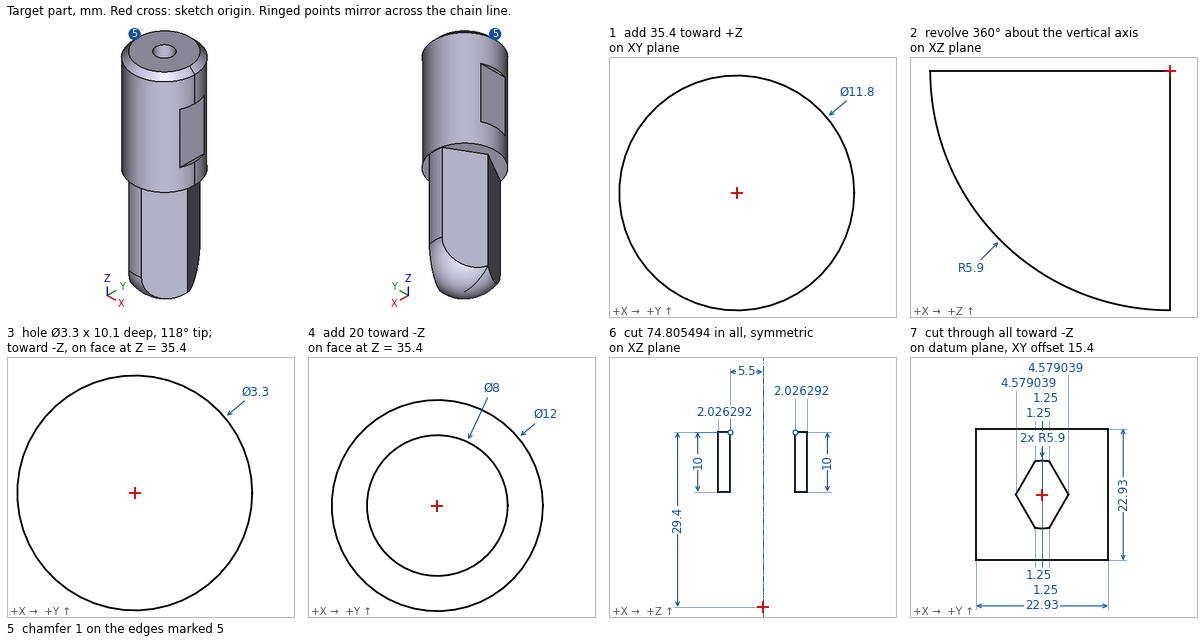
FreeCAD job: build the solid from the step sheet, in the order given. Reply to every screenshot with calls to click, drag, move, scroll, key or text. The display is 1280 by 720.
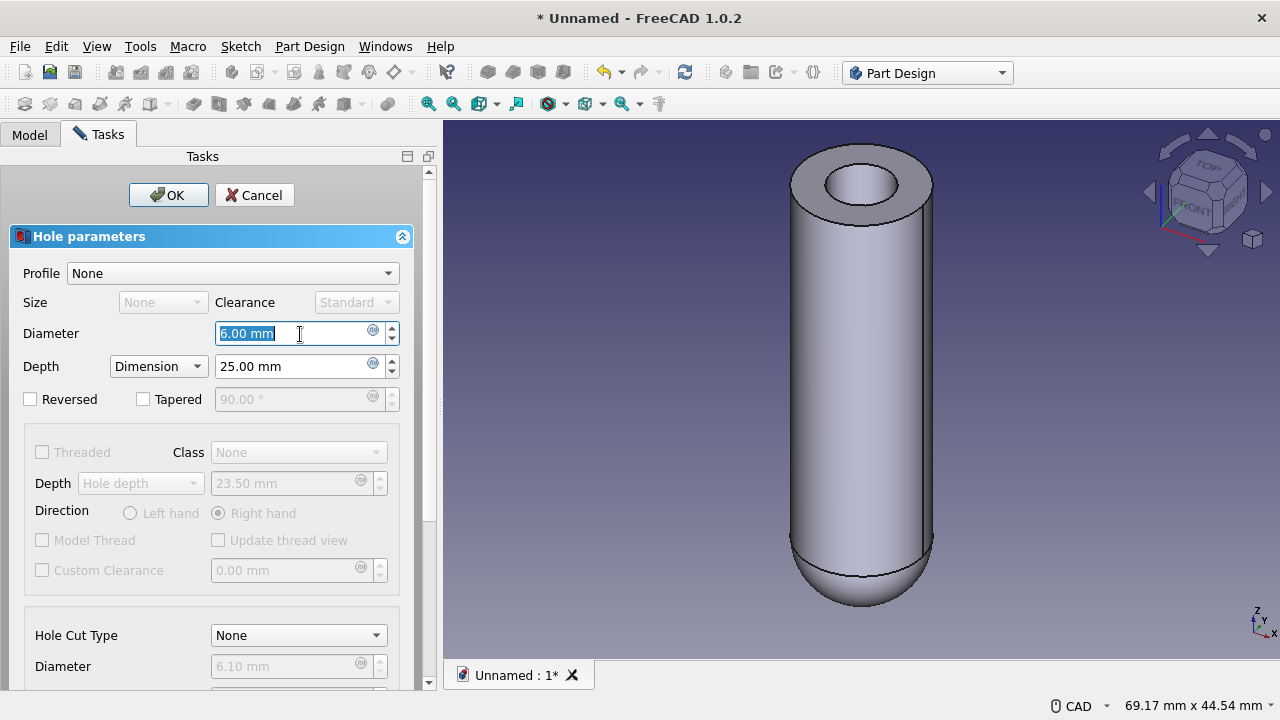
text(3.3)
key(Tab)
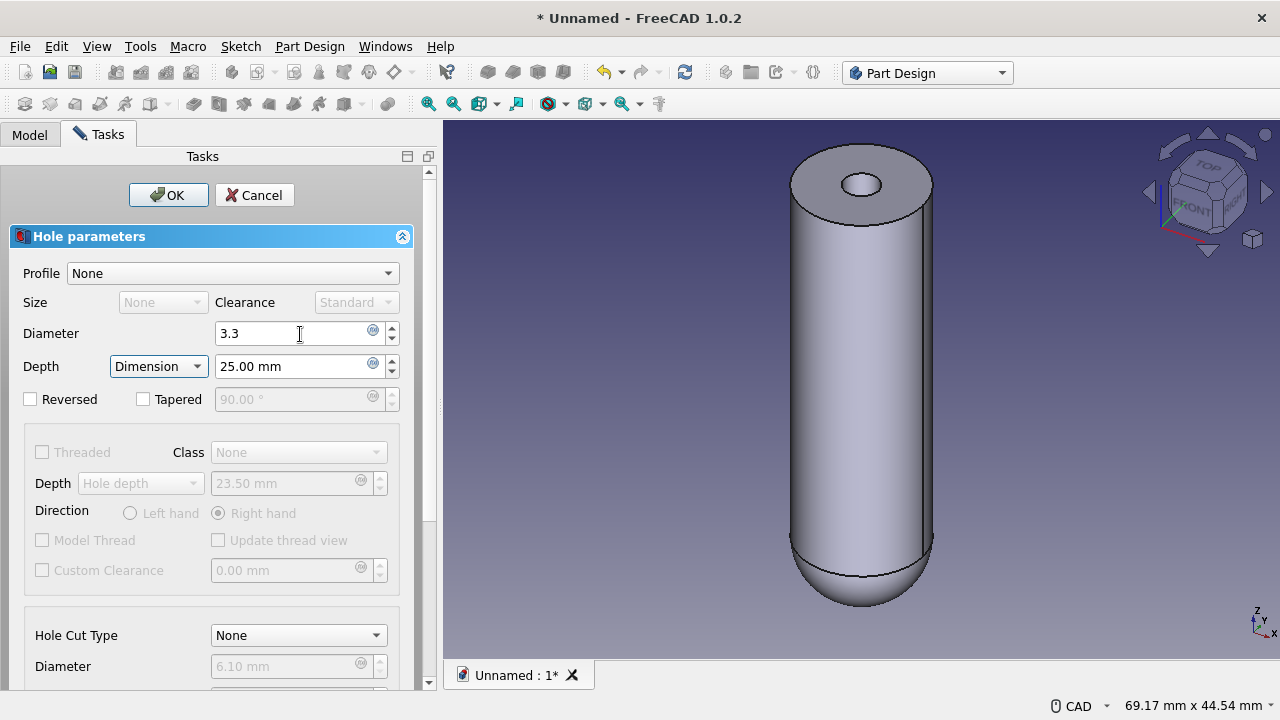
triple_click(300, 366)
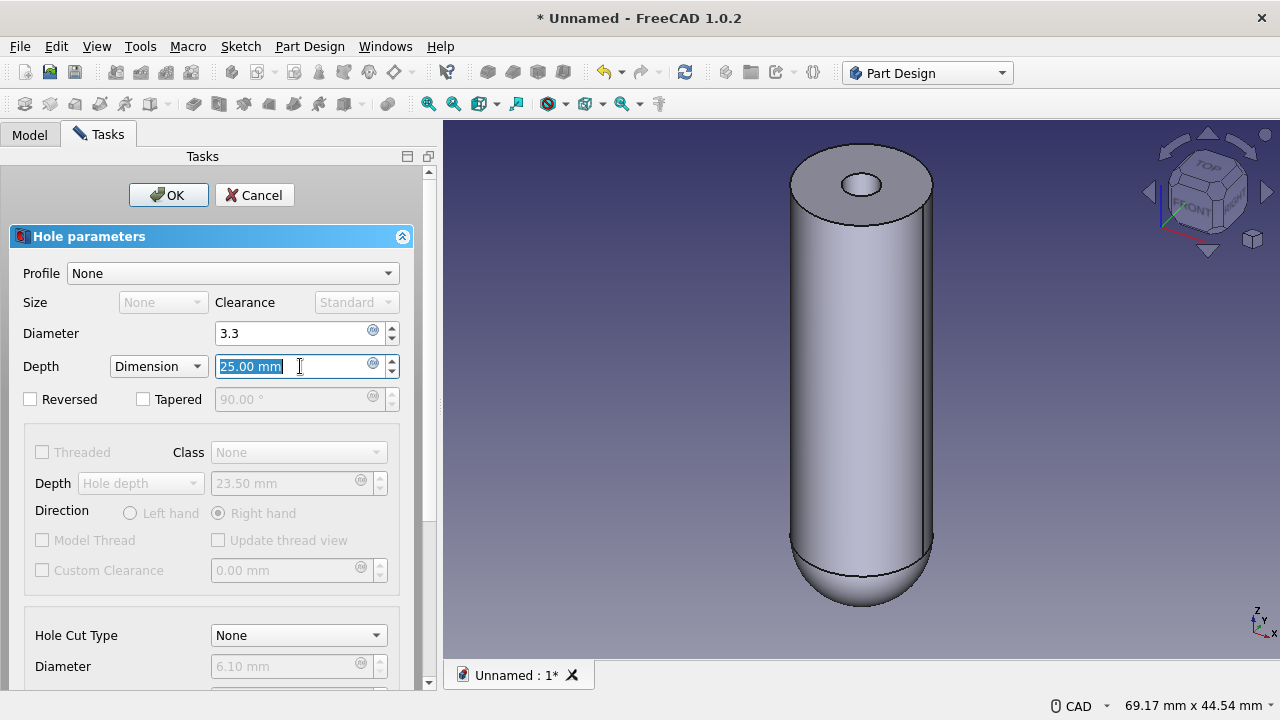
text(10.1)
key(Tab)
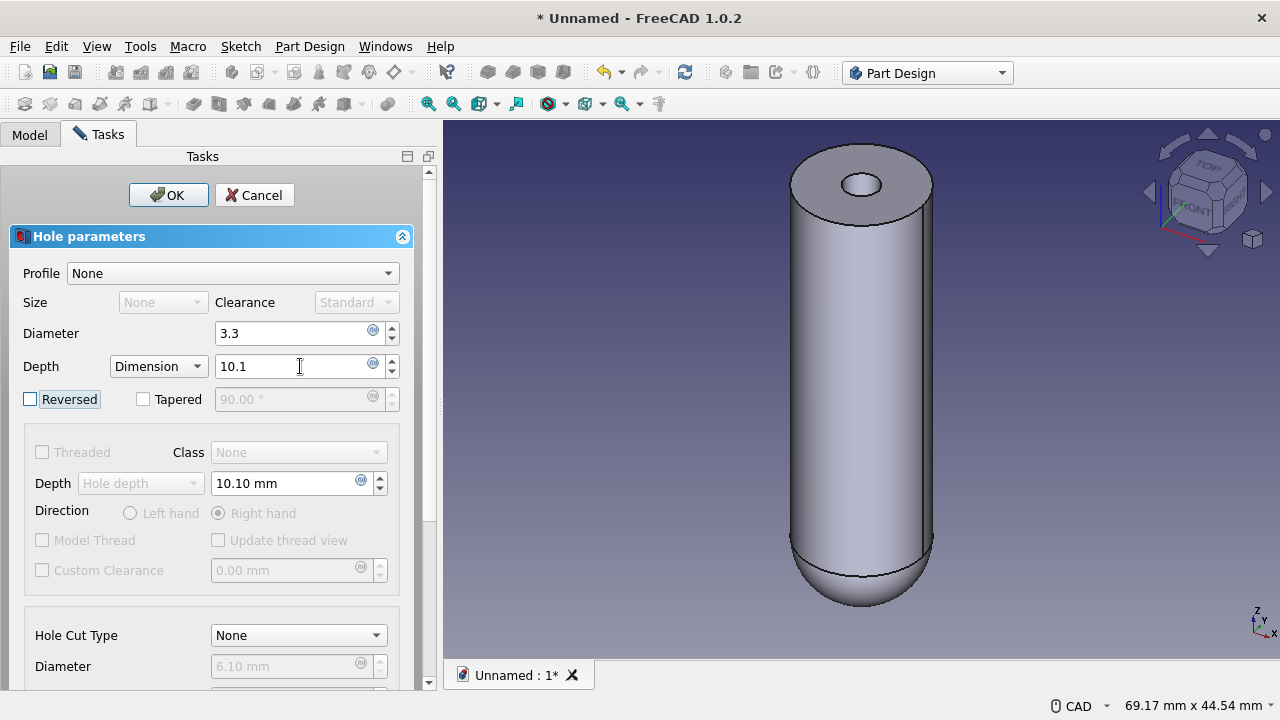
click(169, 195)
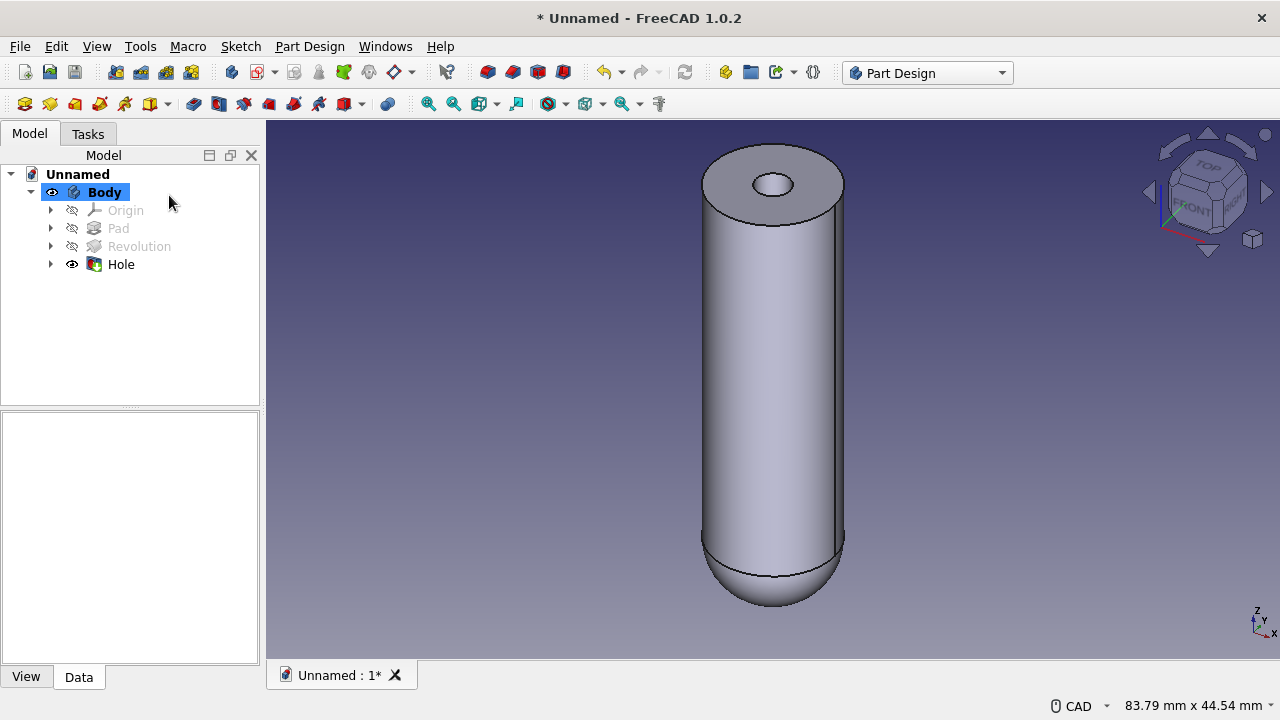
click(819, 185)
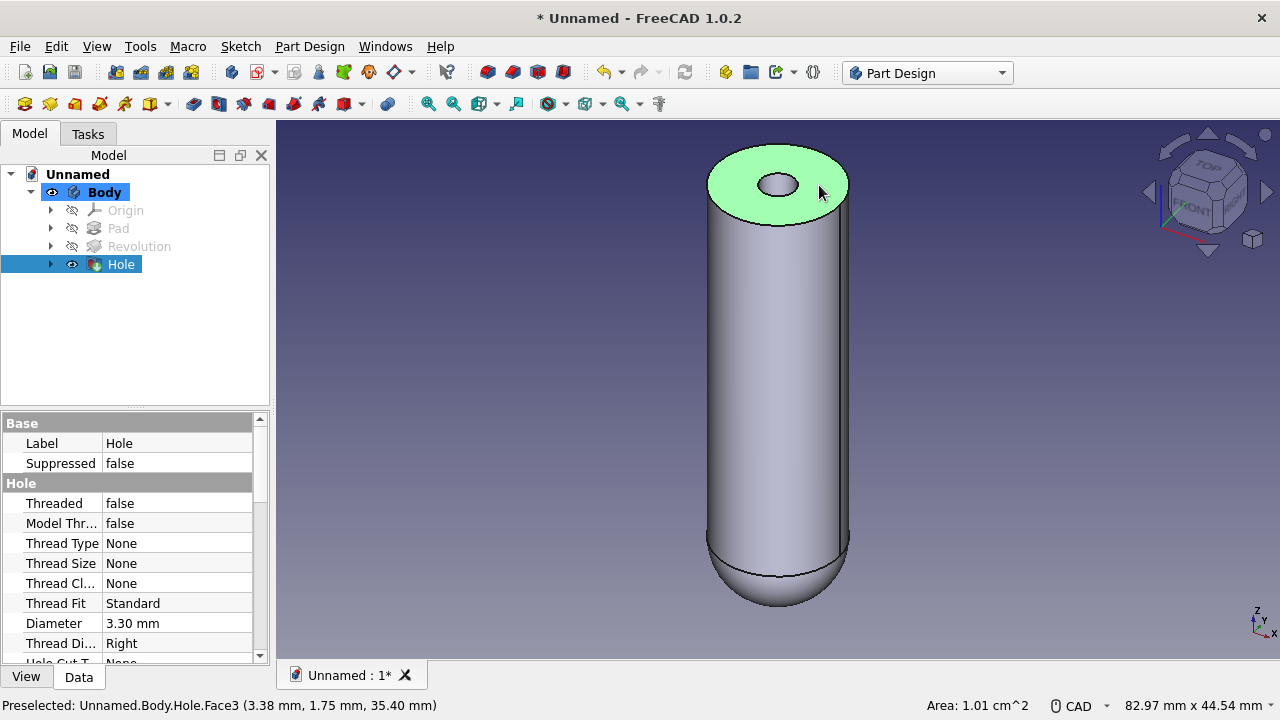
click(256, 72)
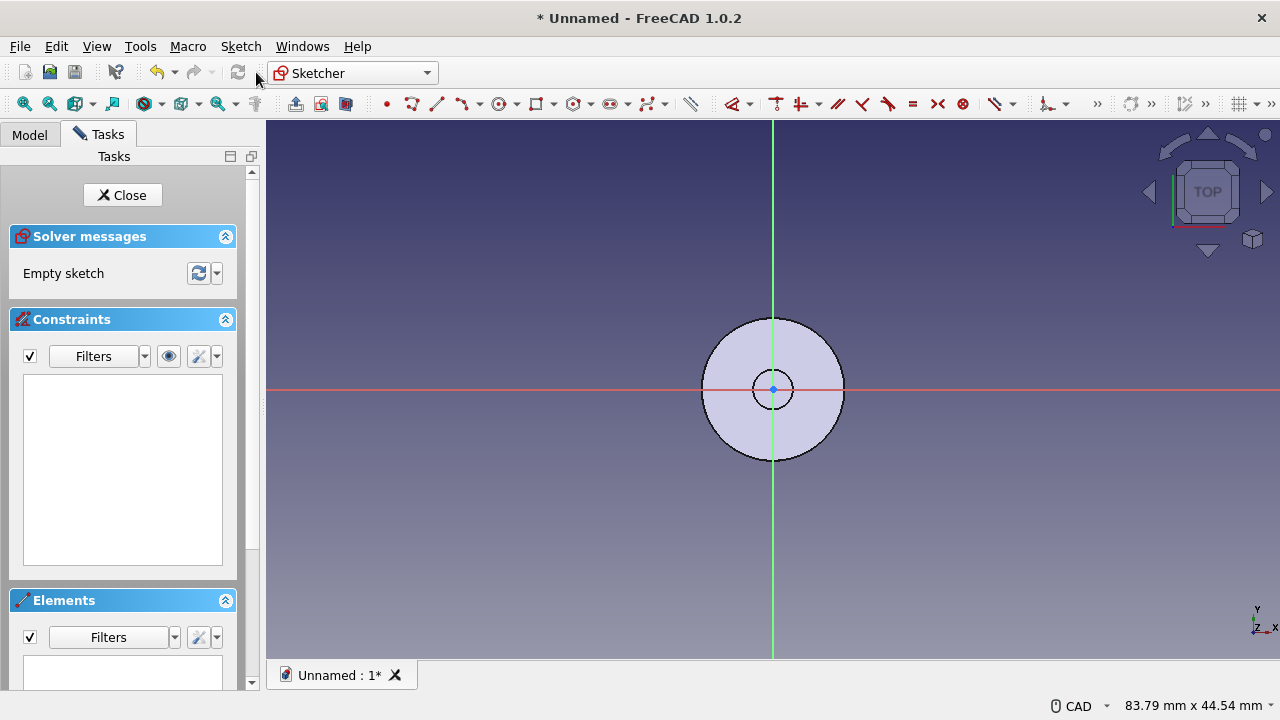
scroll(829, 390, up, 4)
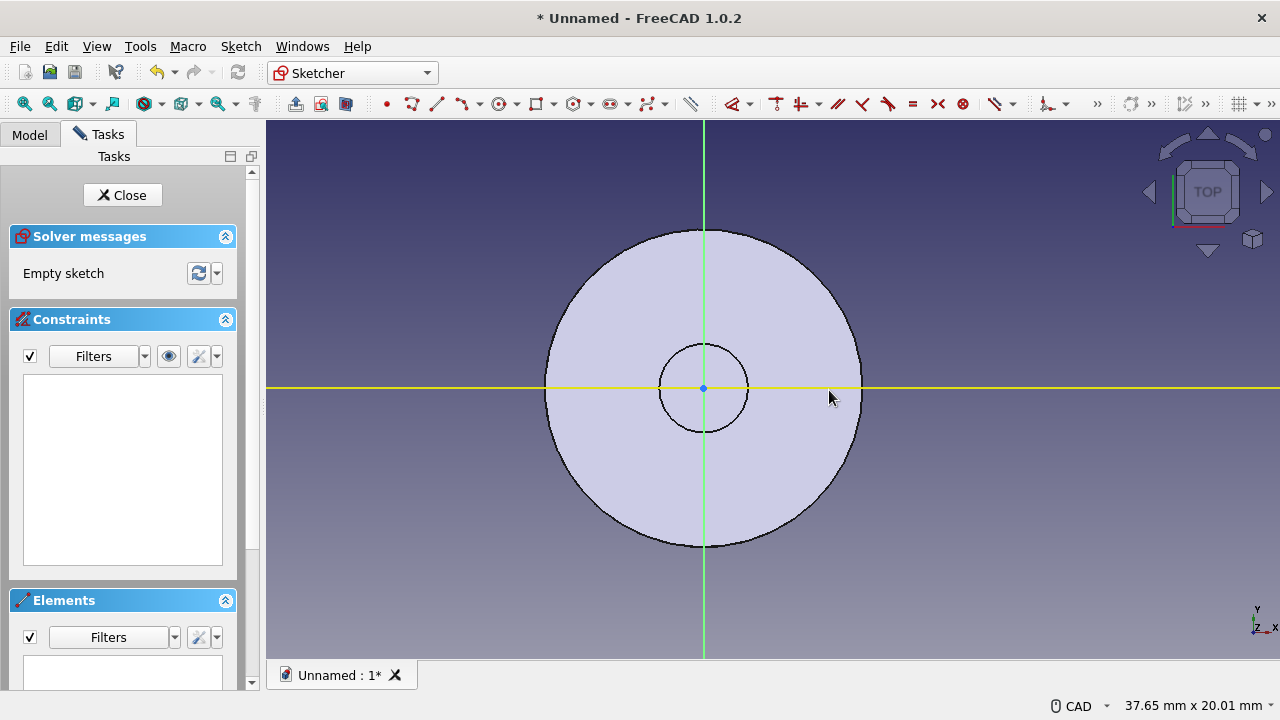
key(g)
key(c)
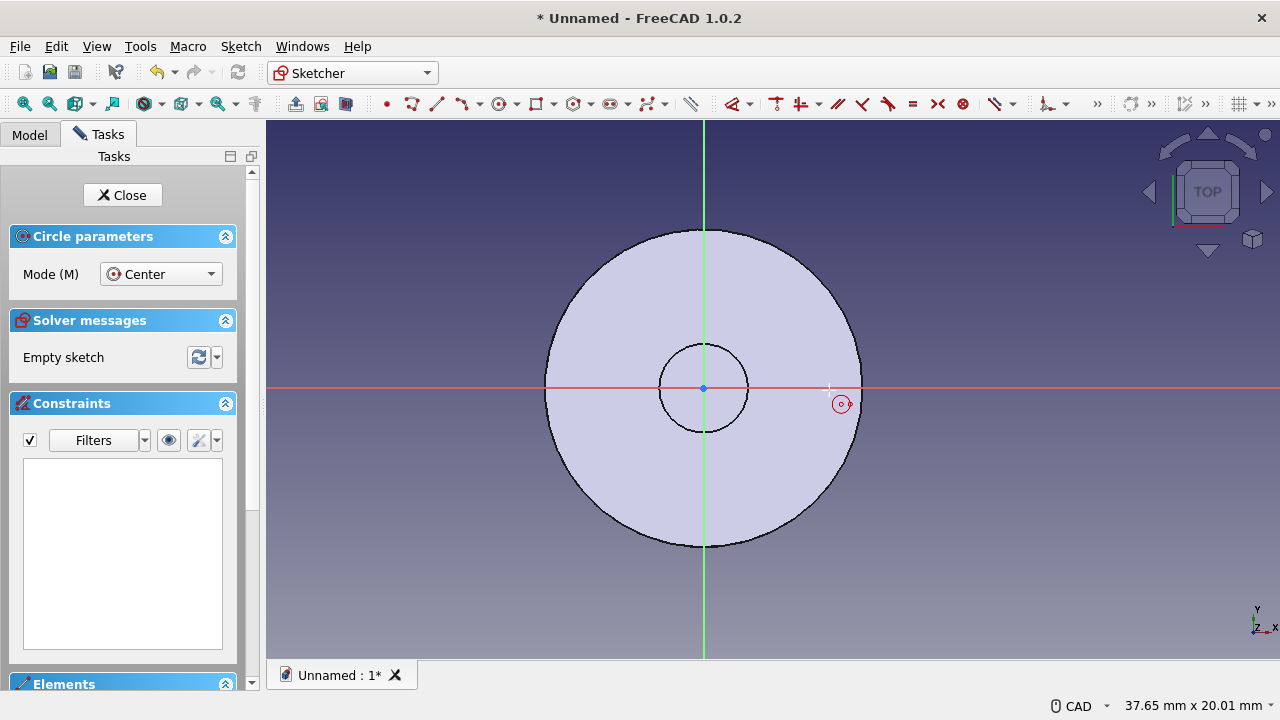
click(704, 388)
move(818, 274)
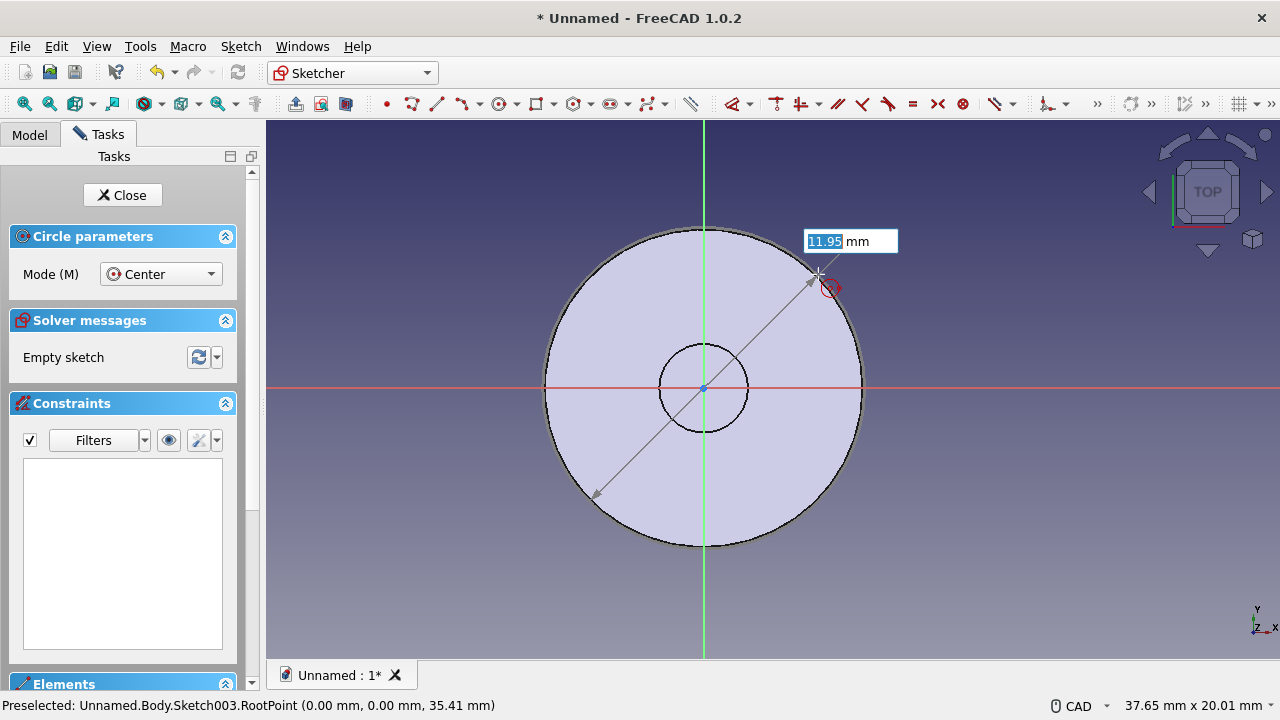
text(12)
key(Return)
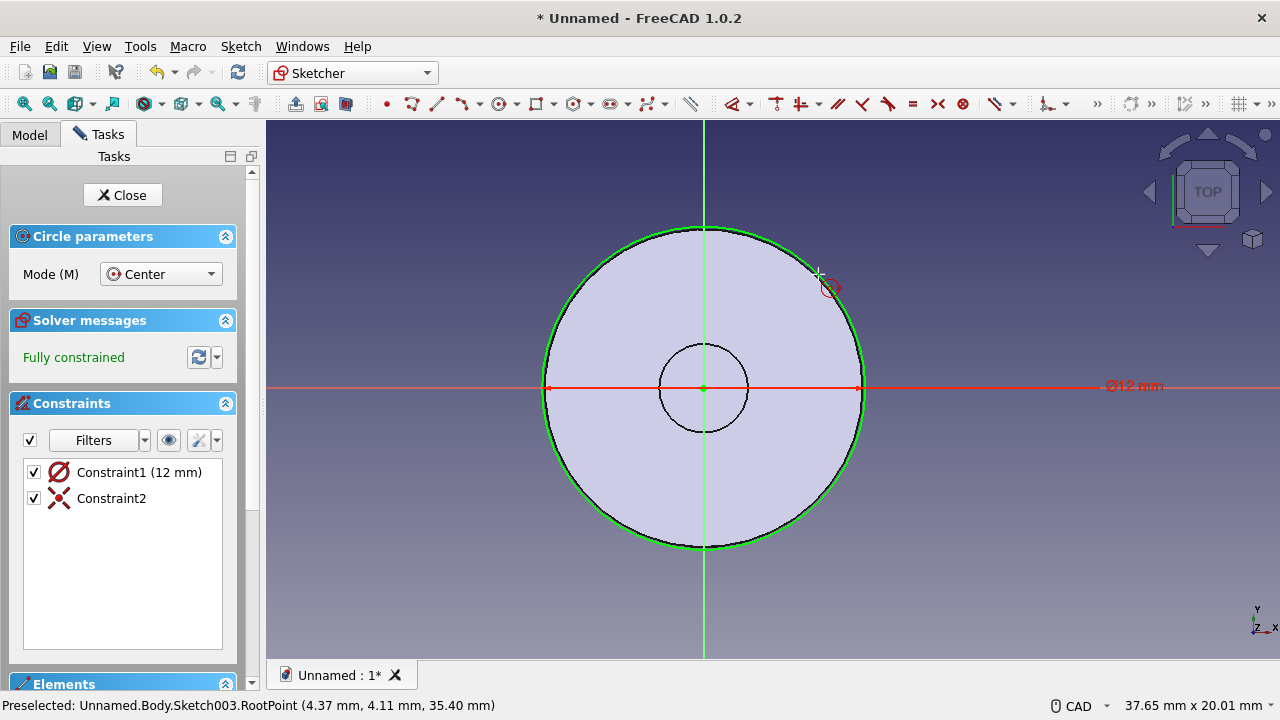
click(704, 388)
move(780, 312)